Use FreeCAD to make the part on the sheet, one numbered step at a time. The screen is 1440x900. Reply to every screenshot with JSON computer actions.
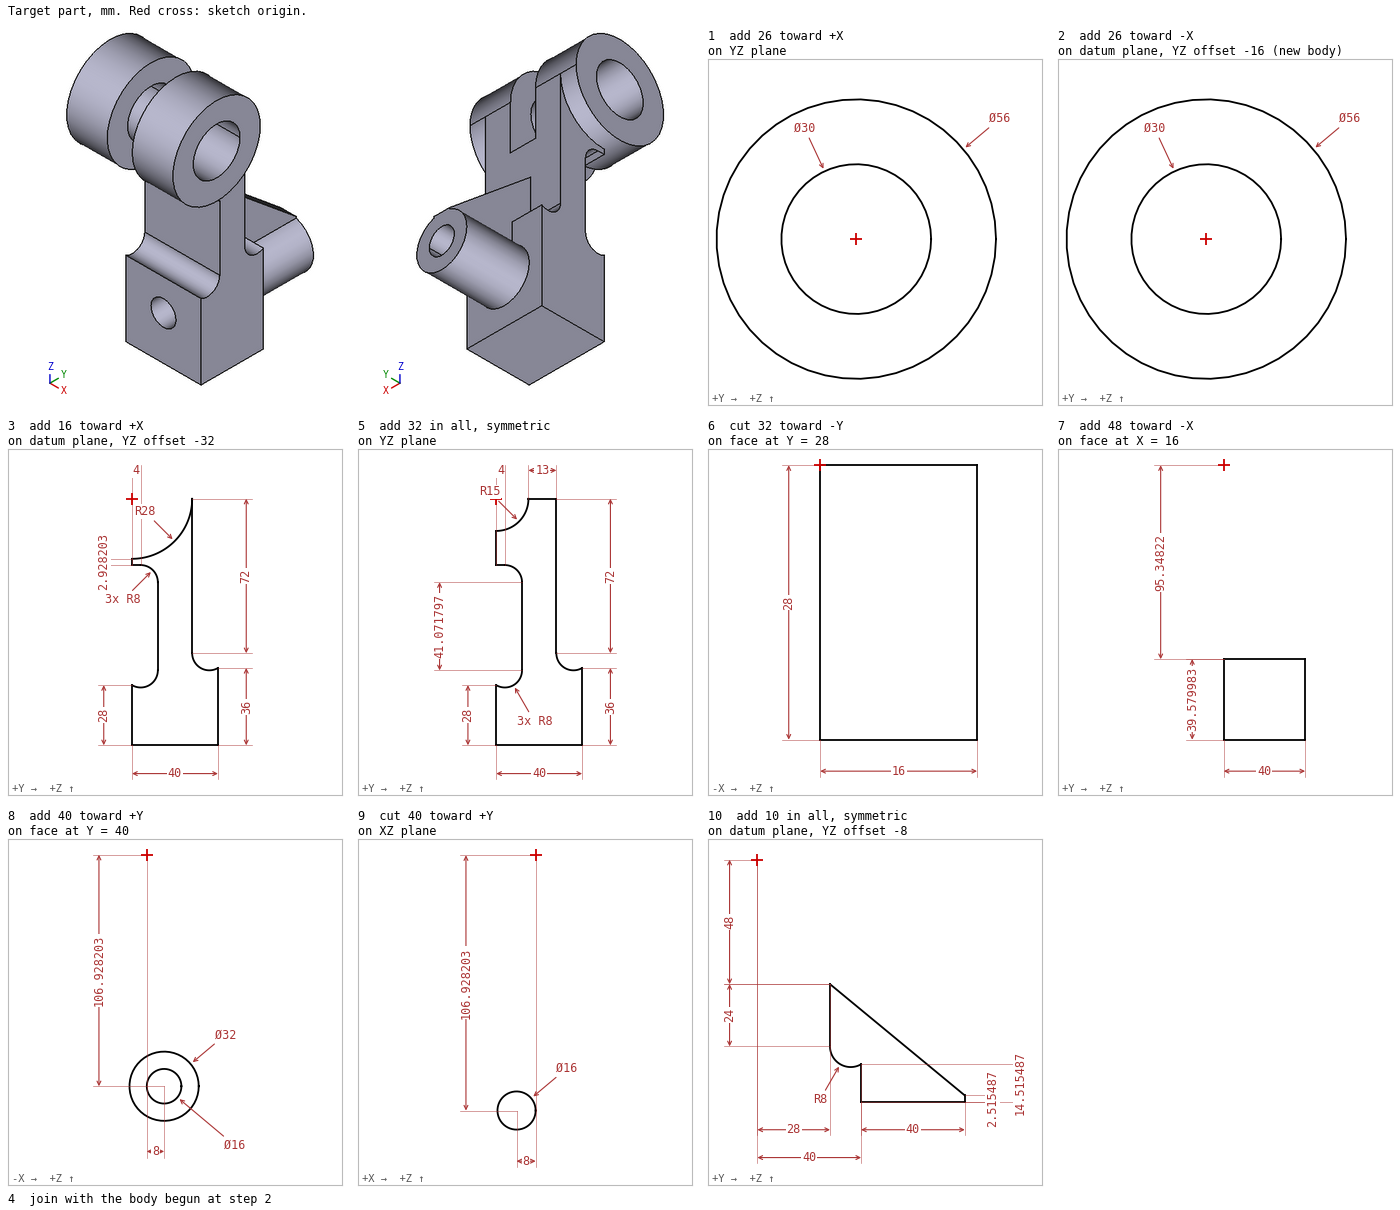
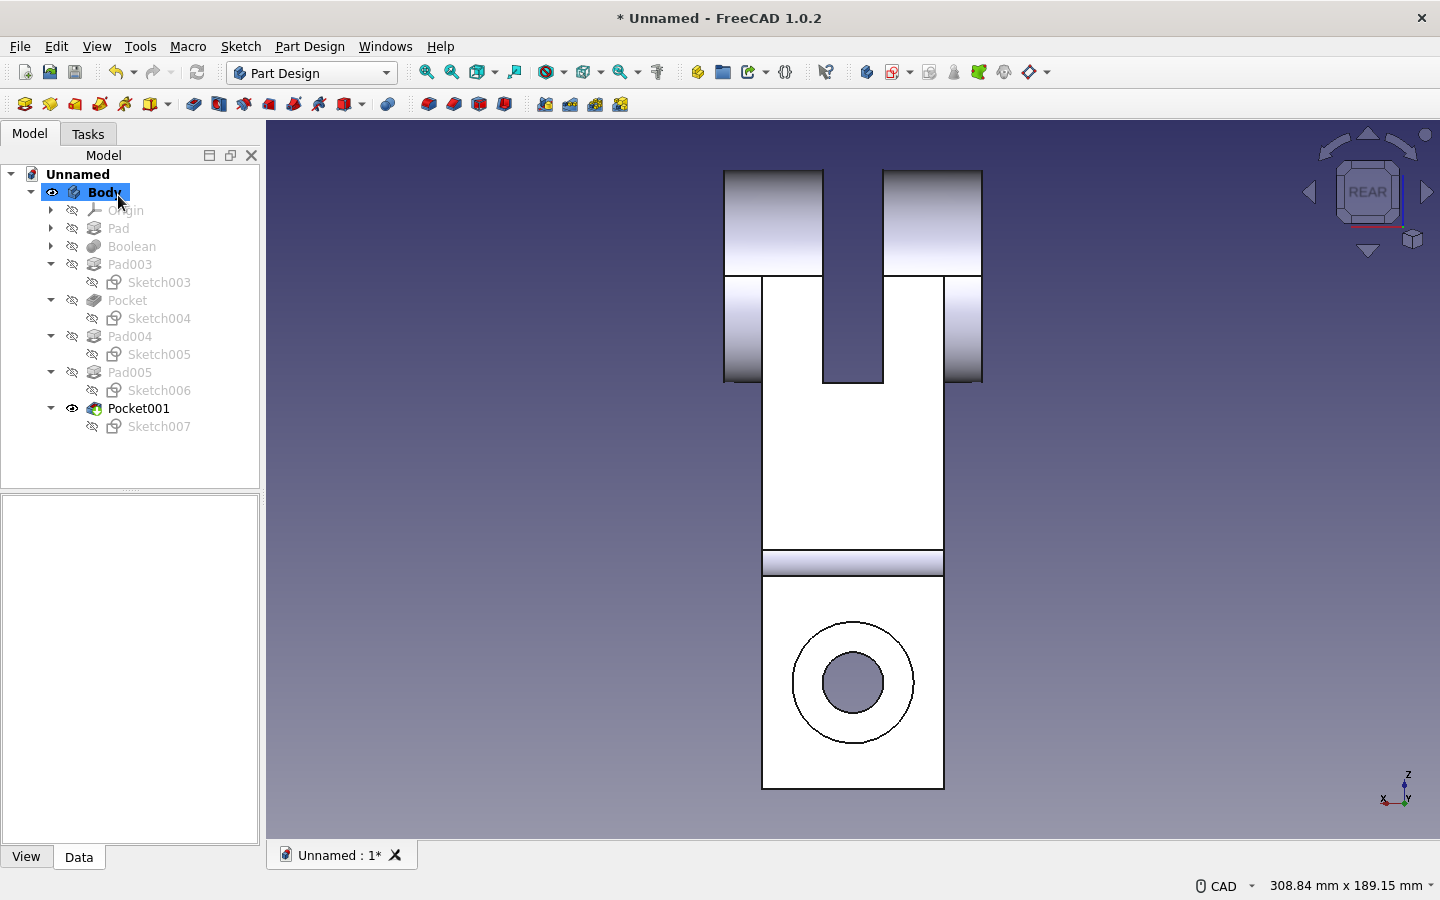
{"action": "left_click", "coordinate": [51, 210]}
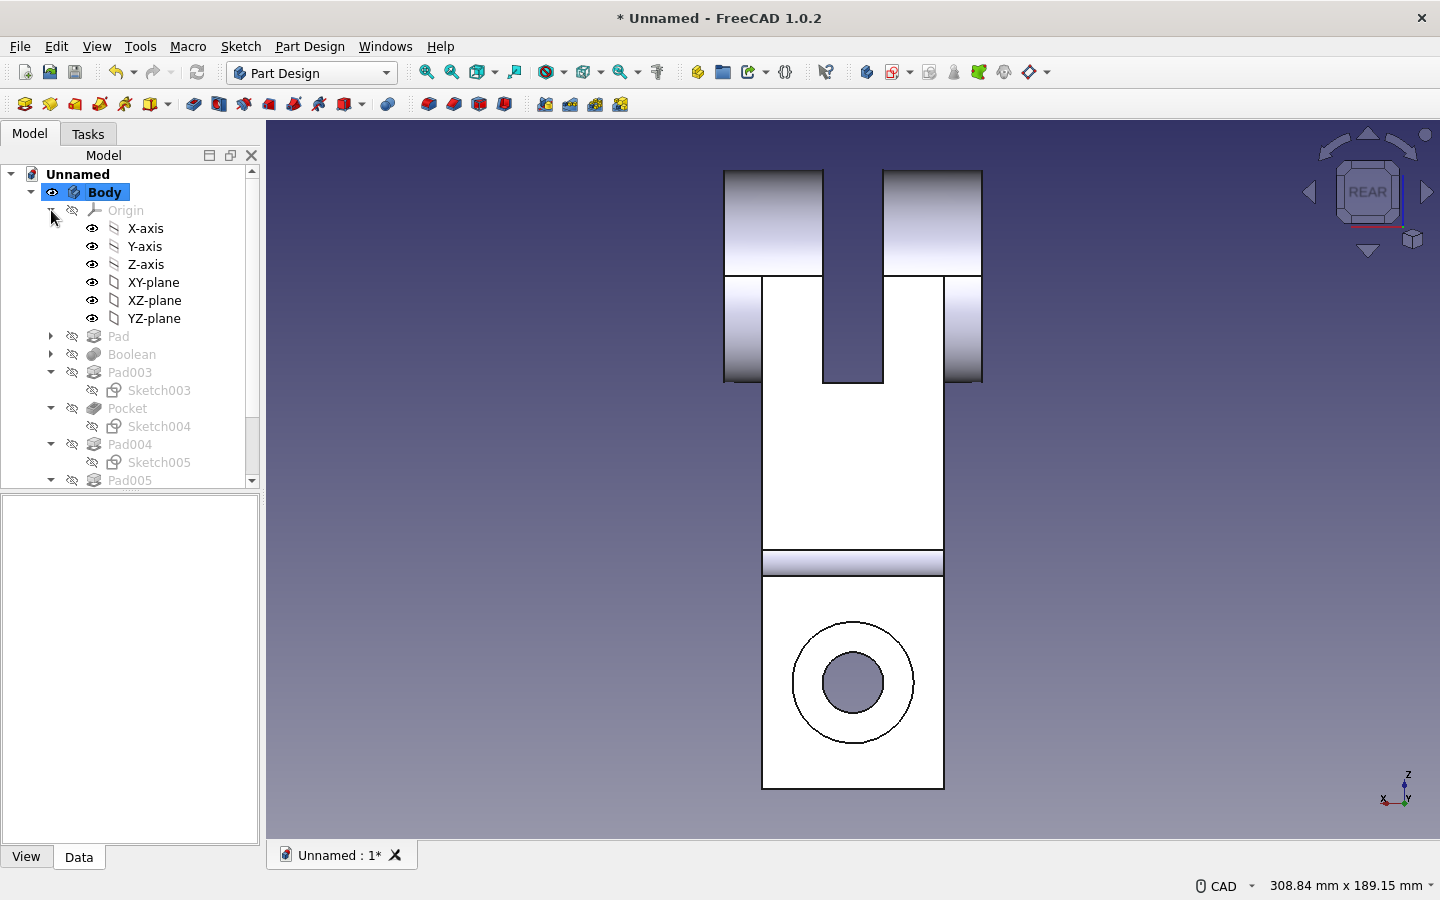
{"action": "left_click", "coordinate": [137, 318]}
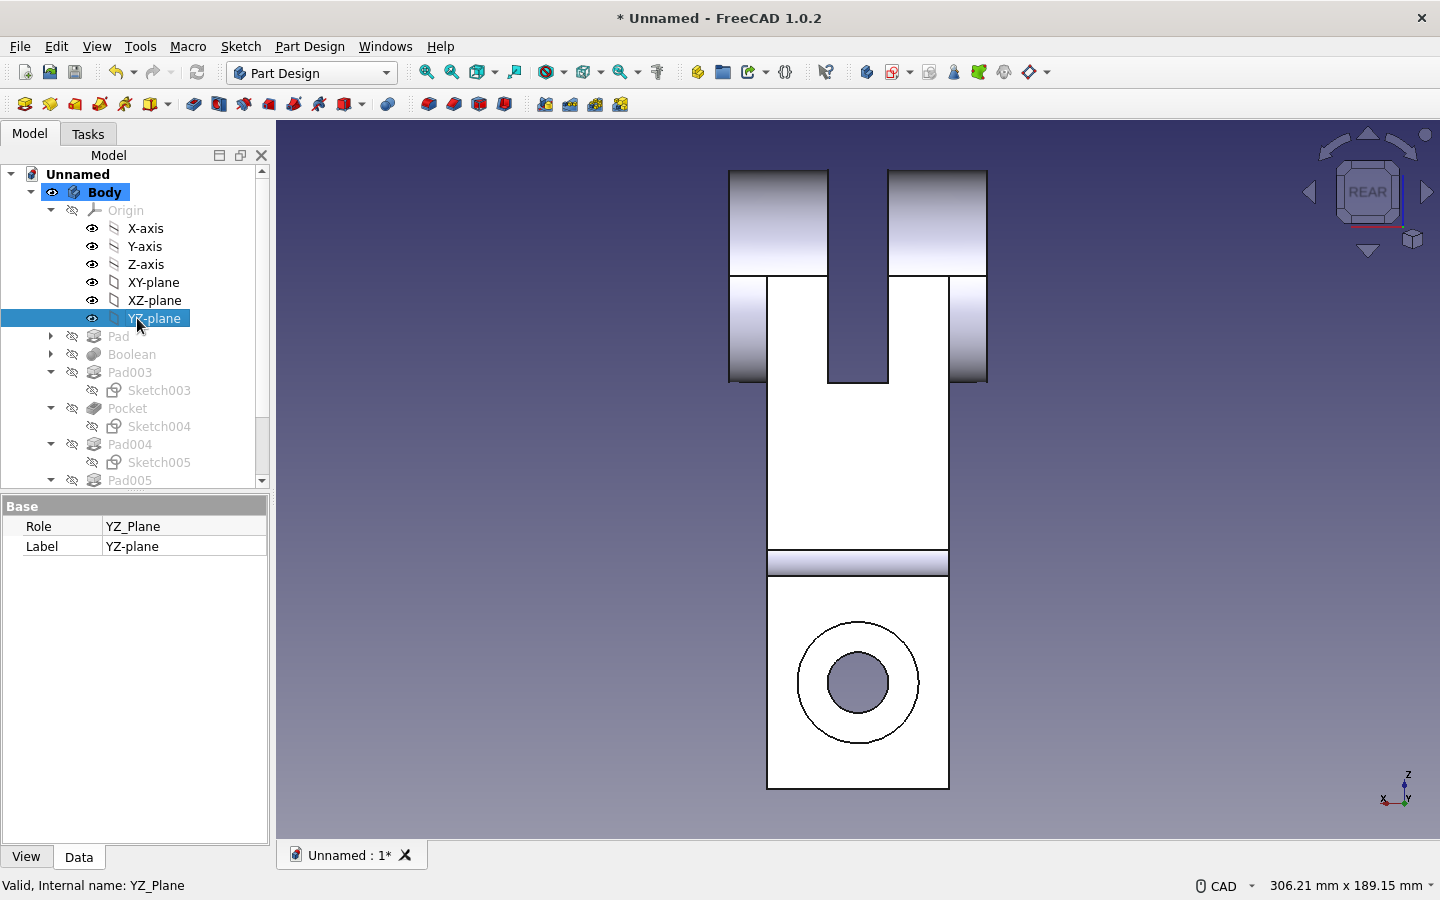
{"action": "left_click", "coordinate": [1028, 72]}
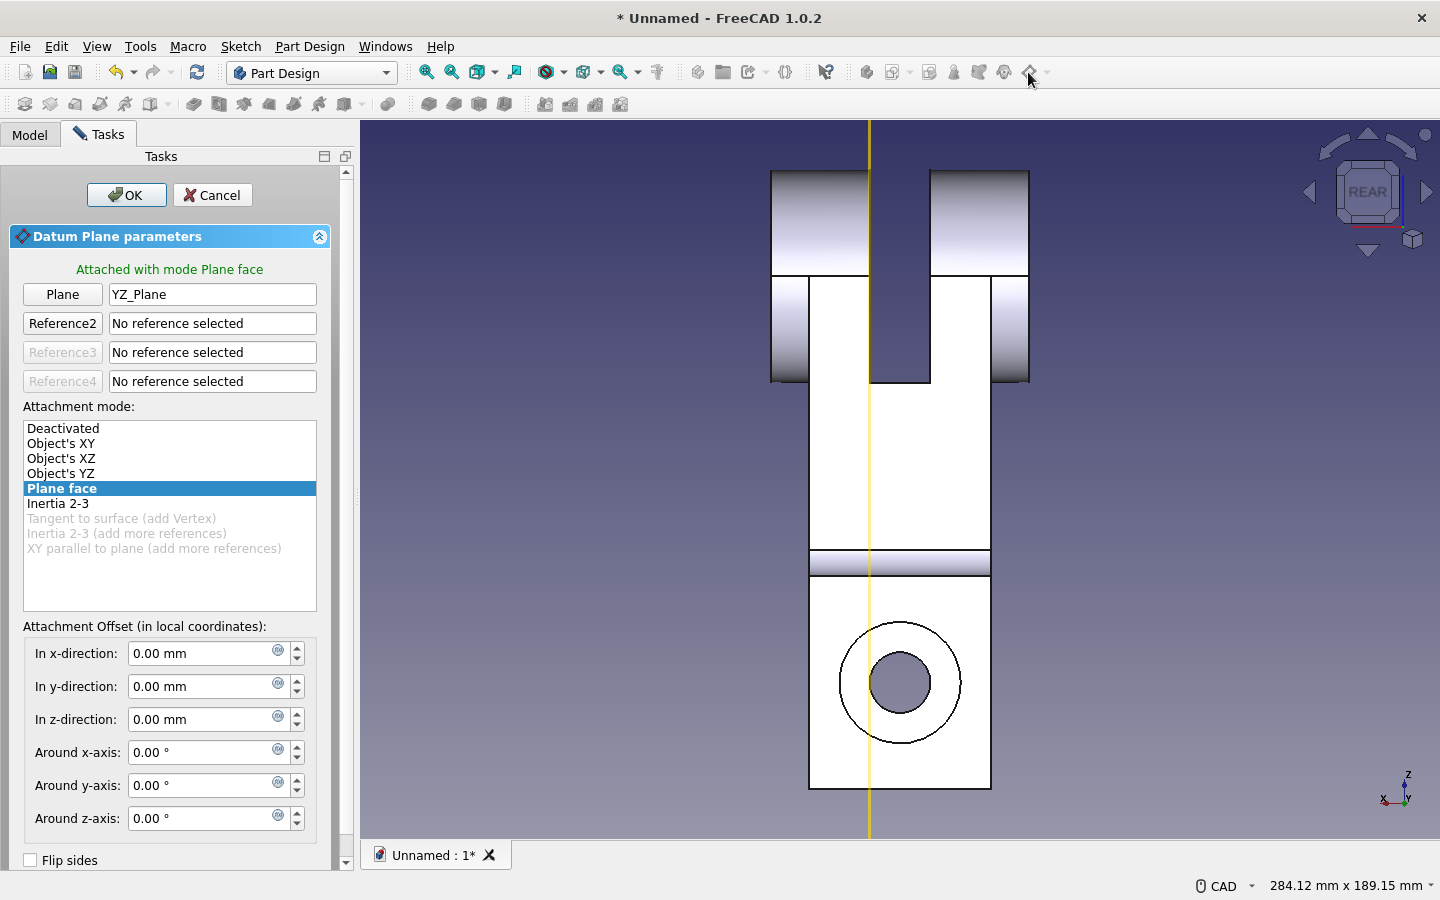
{"action": "triple_click", "coordinate": [210, 720]}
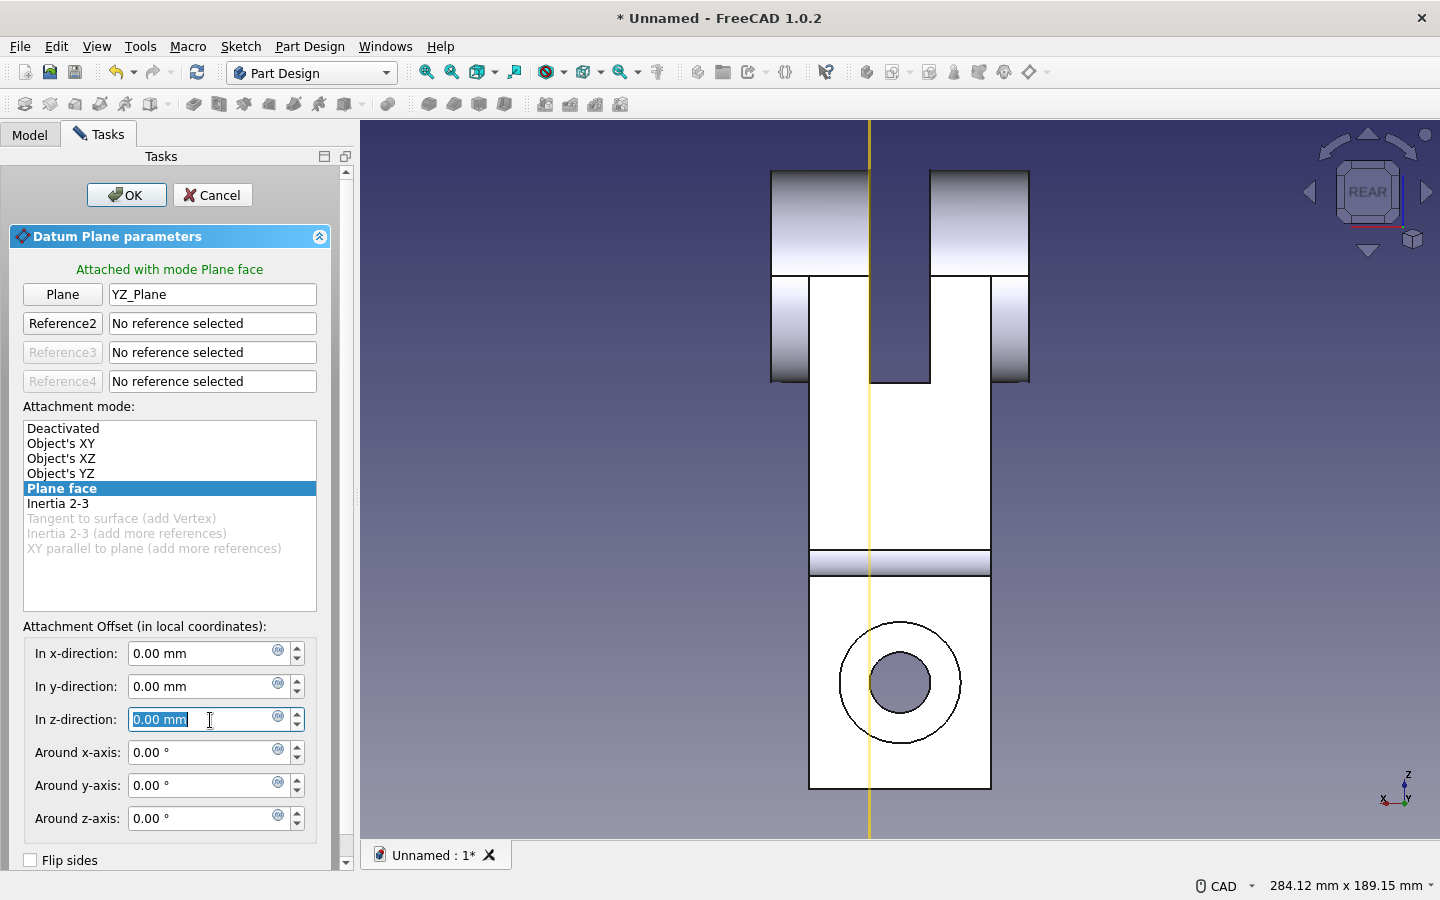
{"action": "type", "text": "-8"}
{"action": "key", "text": "Tab"}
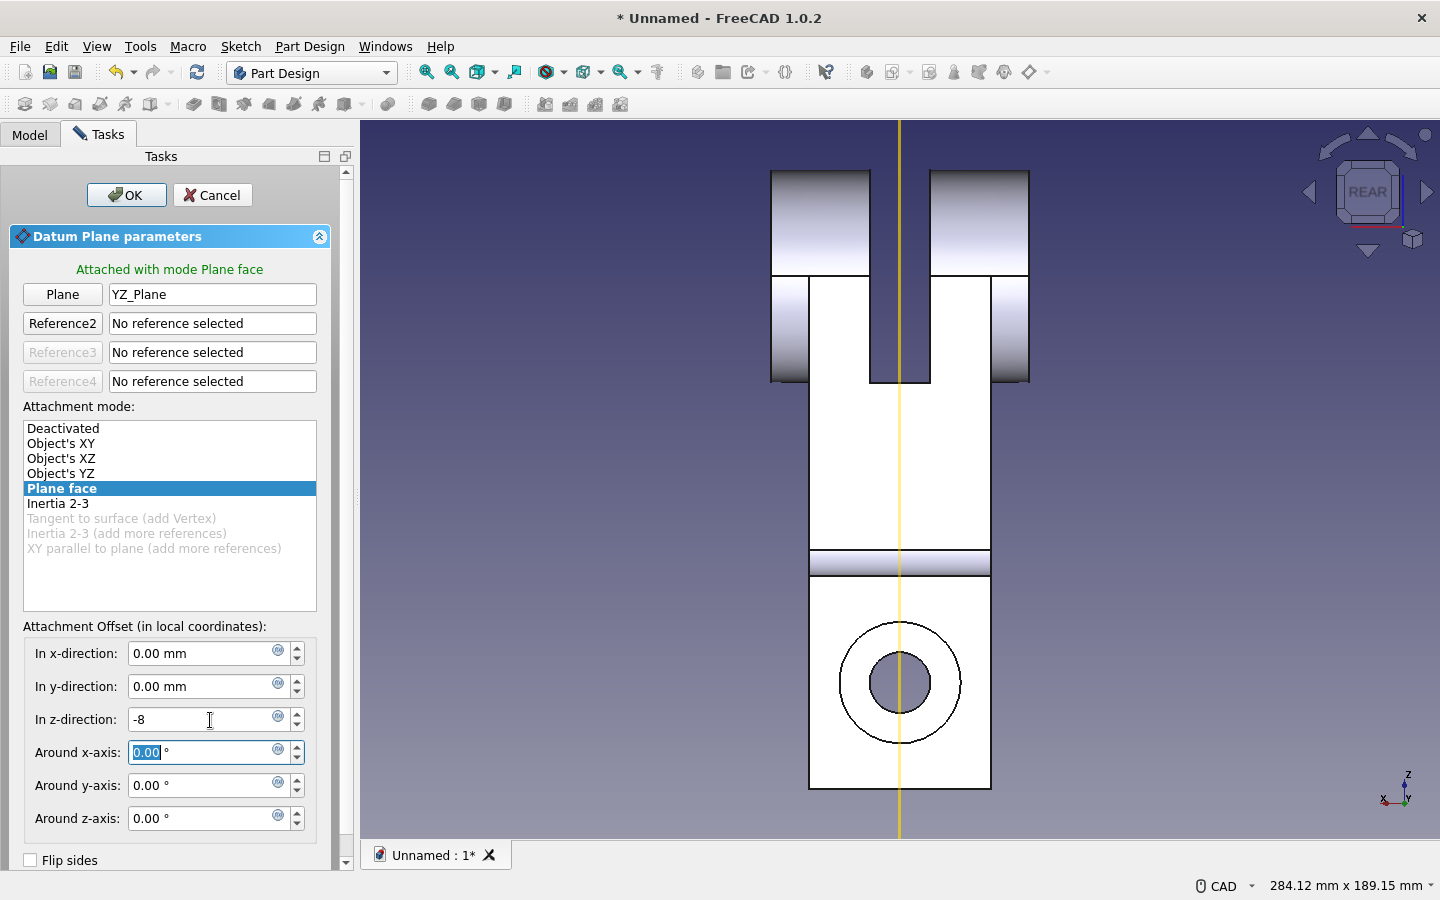
{"action": "left_click", "coordinate": [127, 195]}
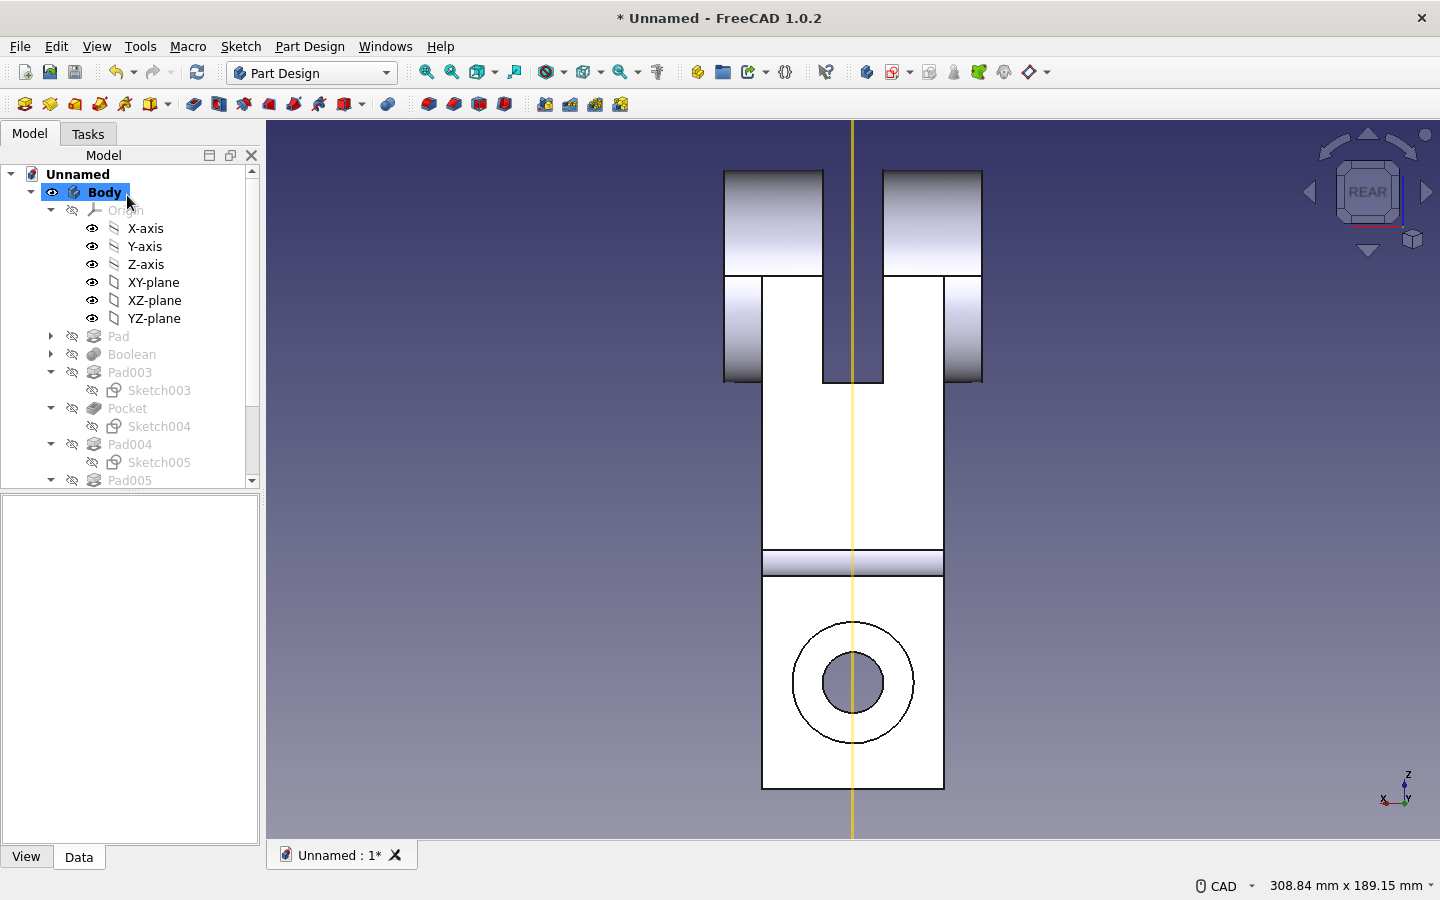
{"action": "scroll", "coordinate": [101, 332], "scroll_direction": "down", "scroll_amount": 3}